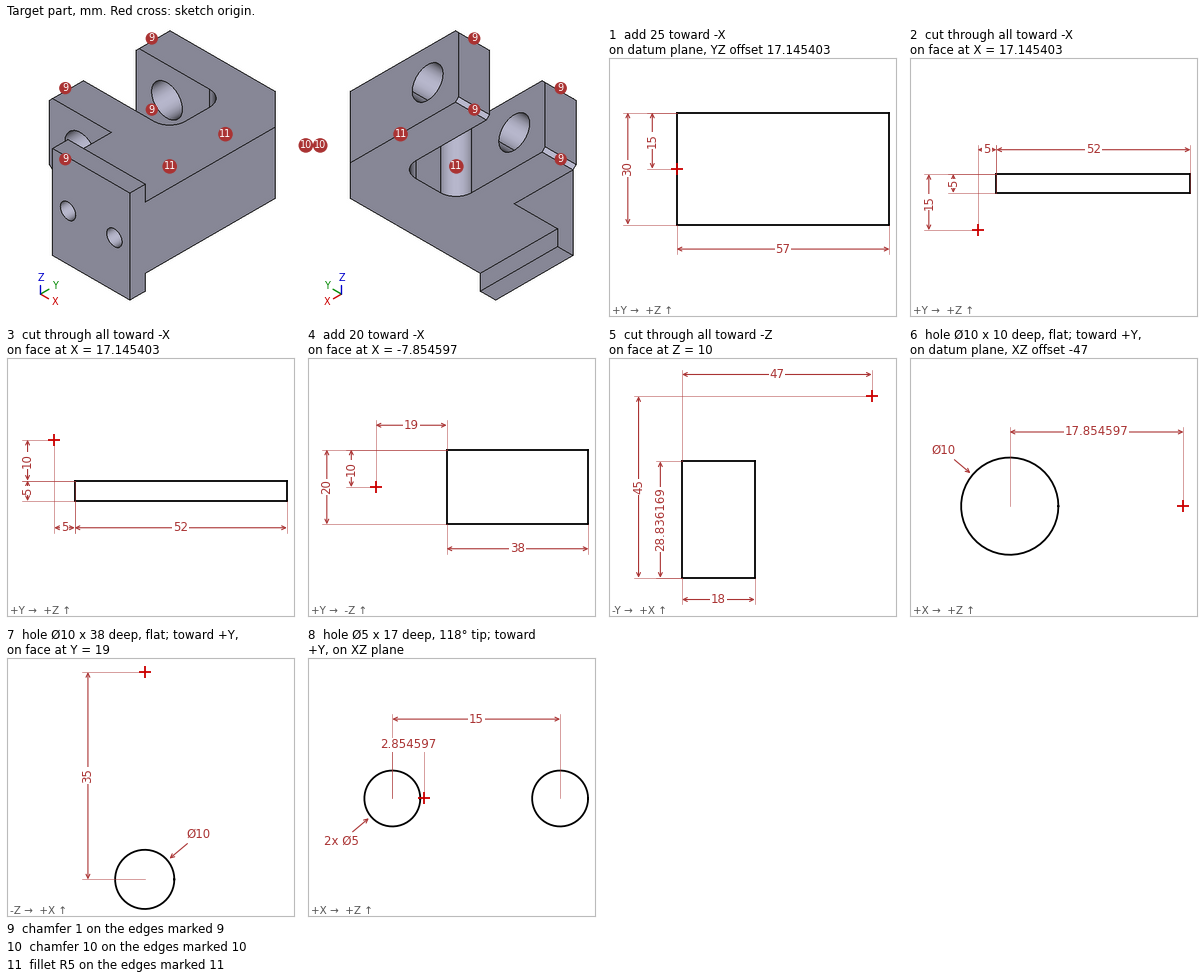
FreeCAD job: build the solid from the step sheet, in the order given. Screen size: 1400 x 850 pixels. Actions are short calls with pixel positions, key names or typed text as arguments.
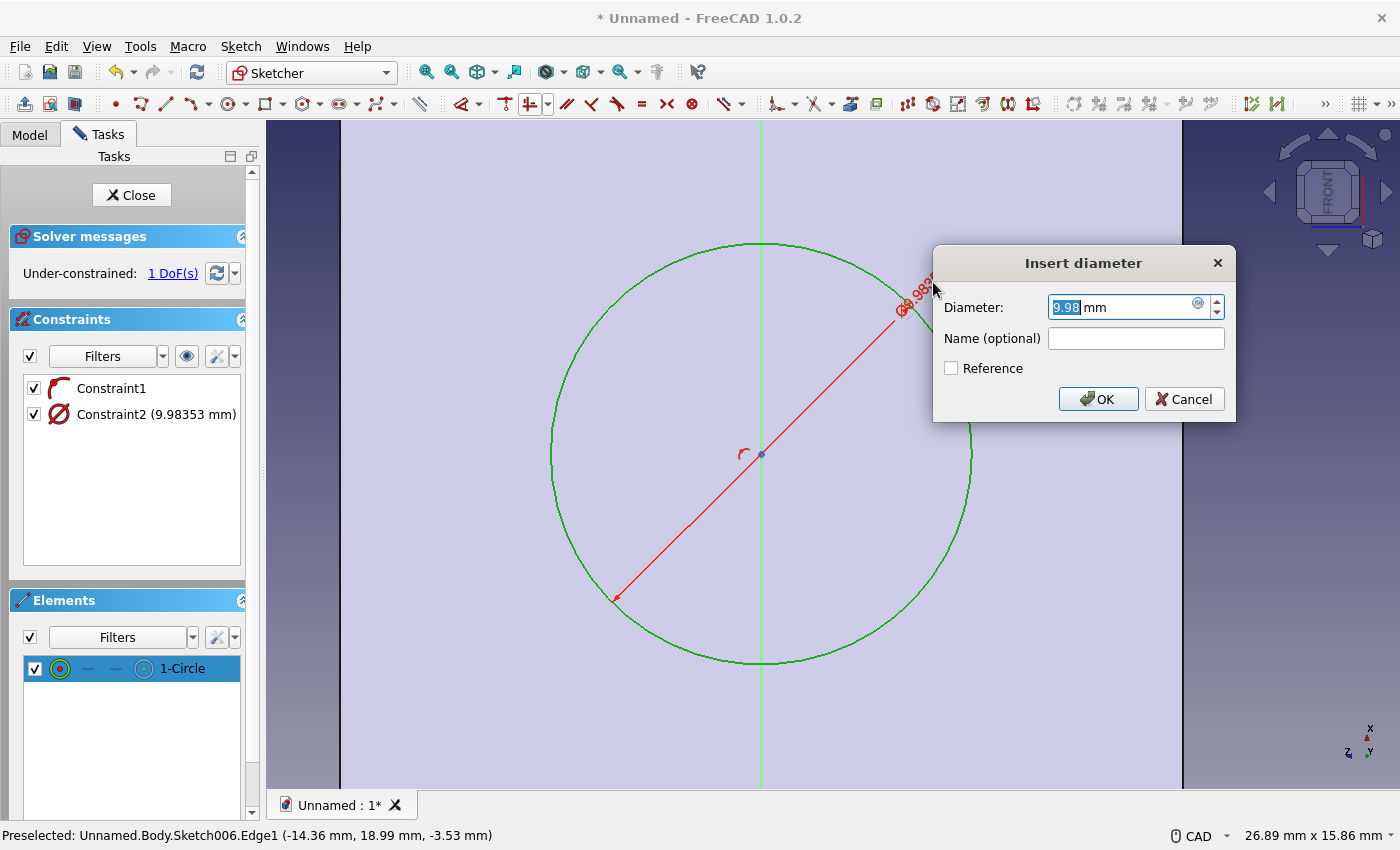
text(10)
key(Return)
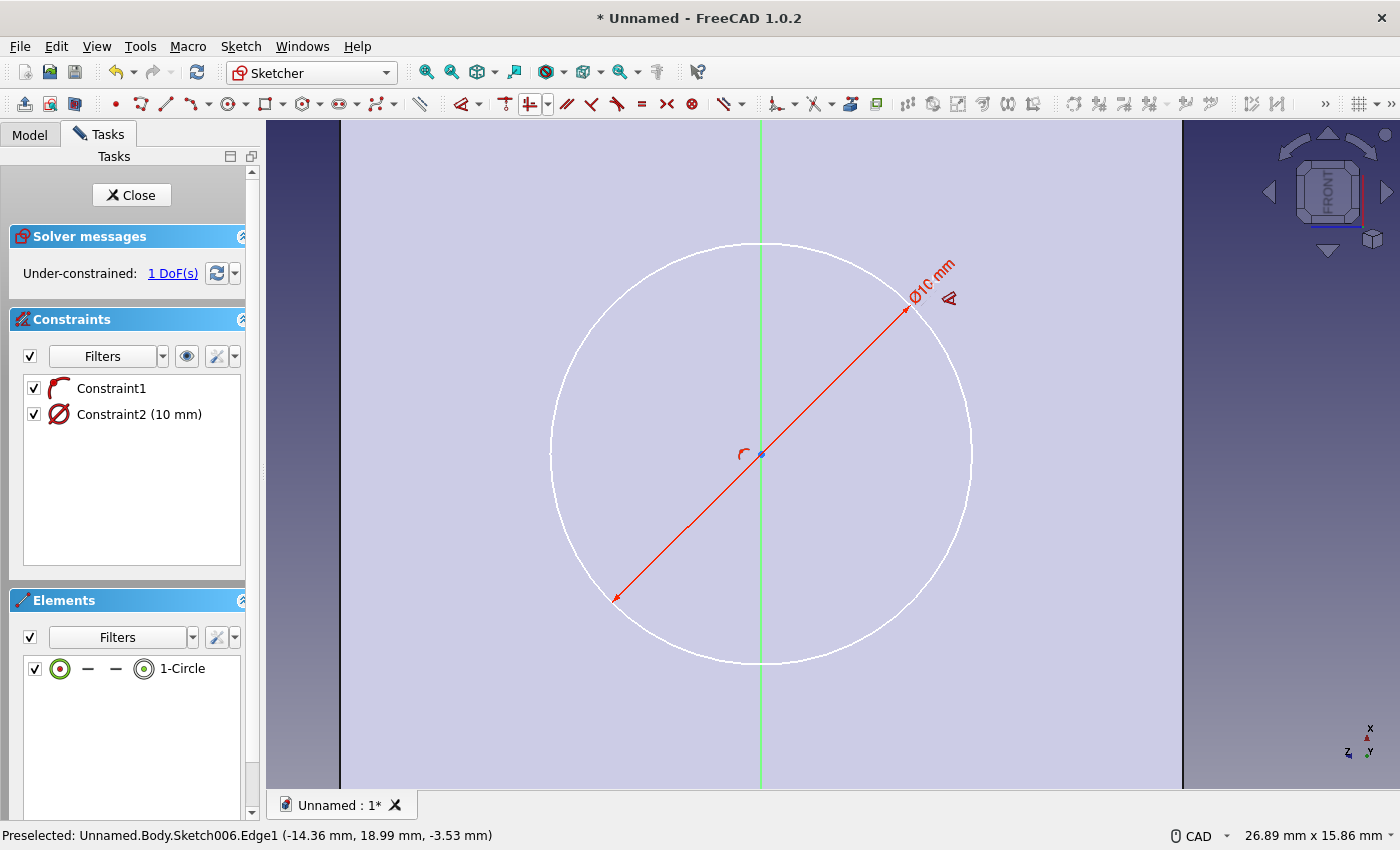
click(761, 454)
click(795, 301)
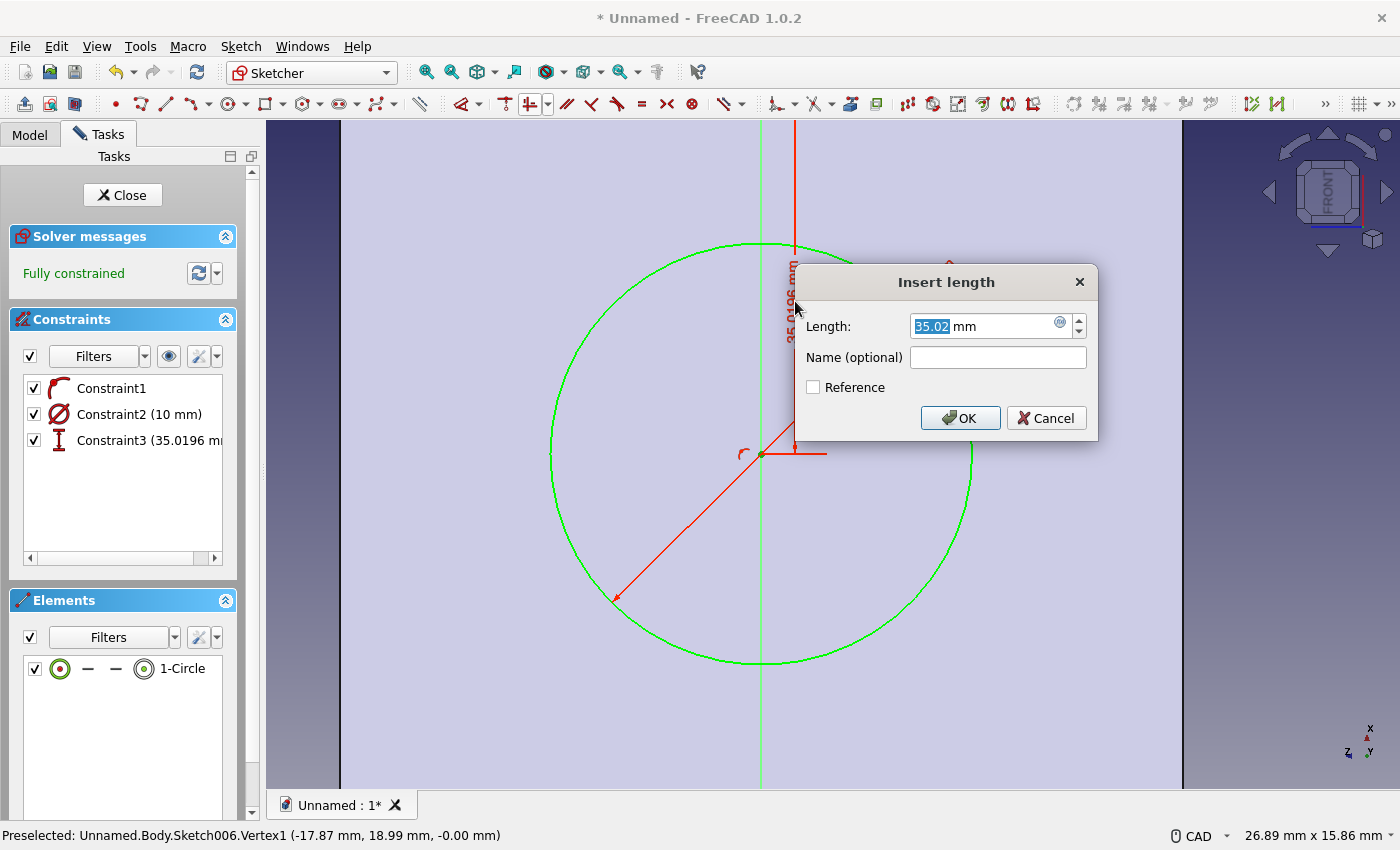
text(35)
key(Return)
key(Escape)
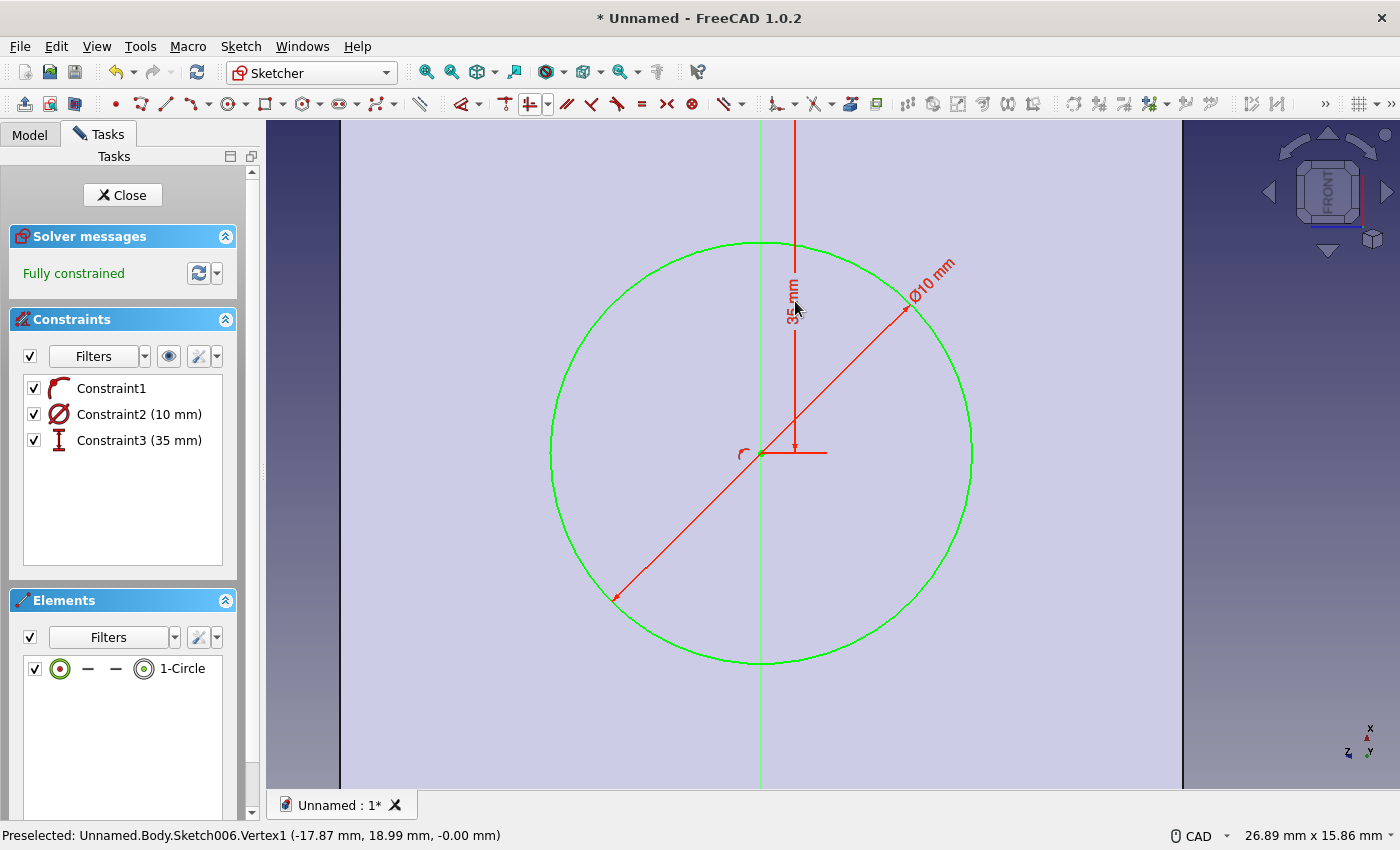
click(123, 195)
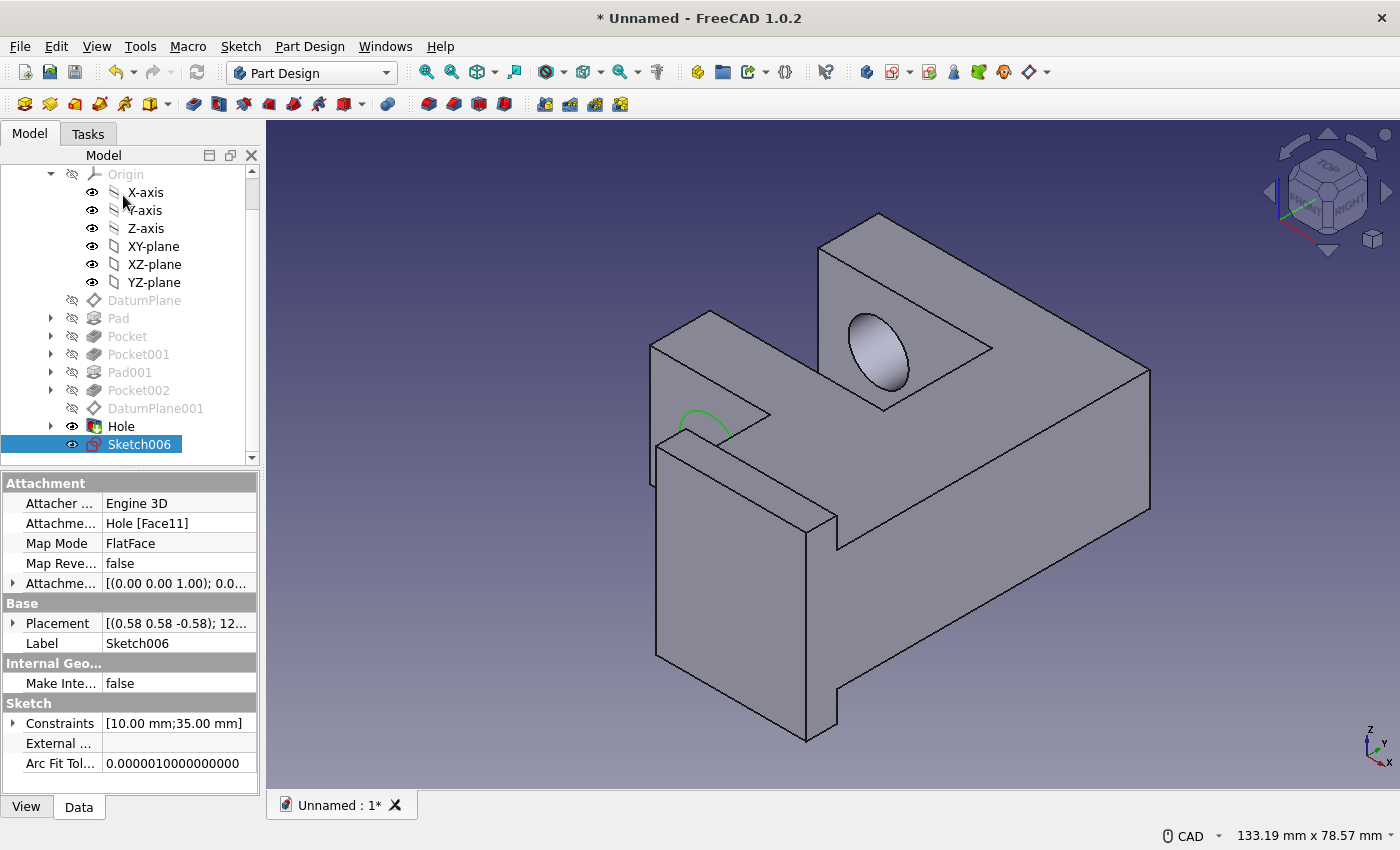
click(219, 104)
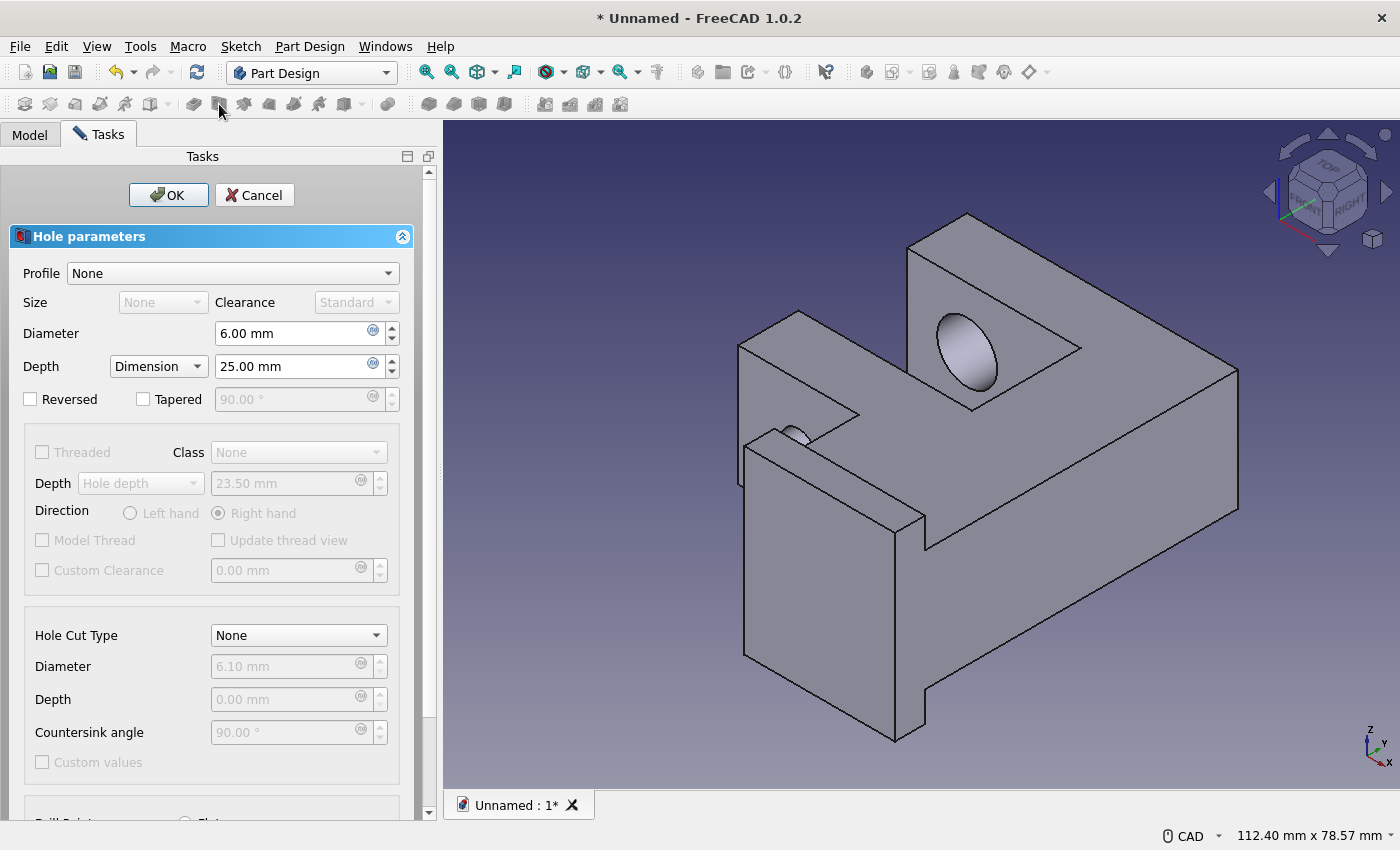
triple_click(300, 334)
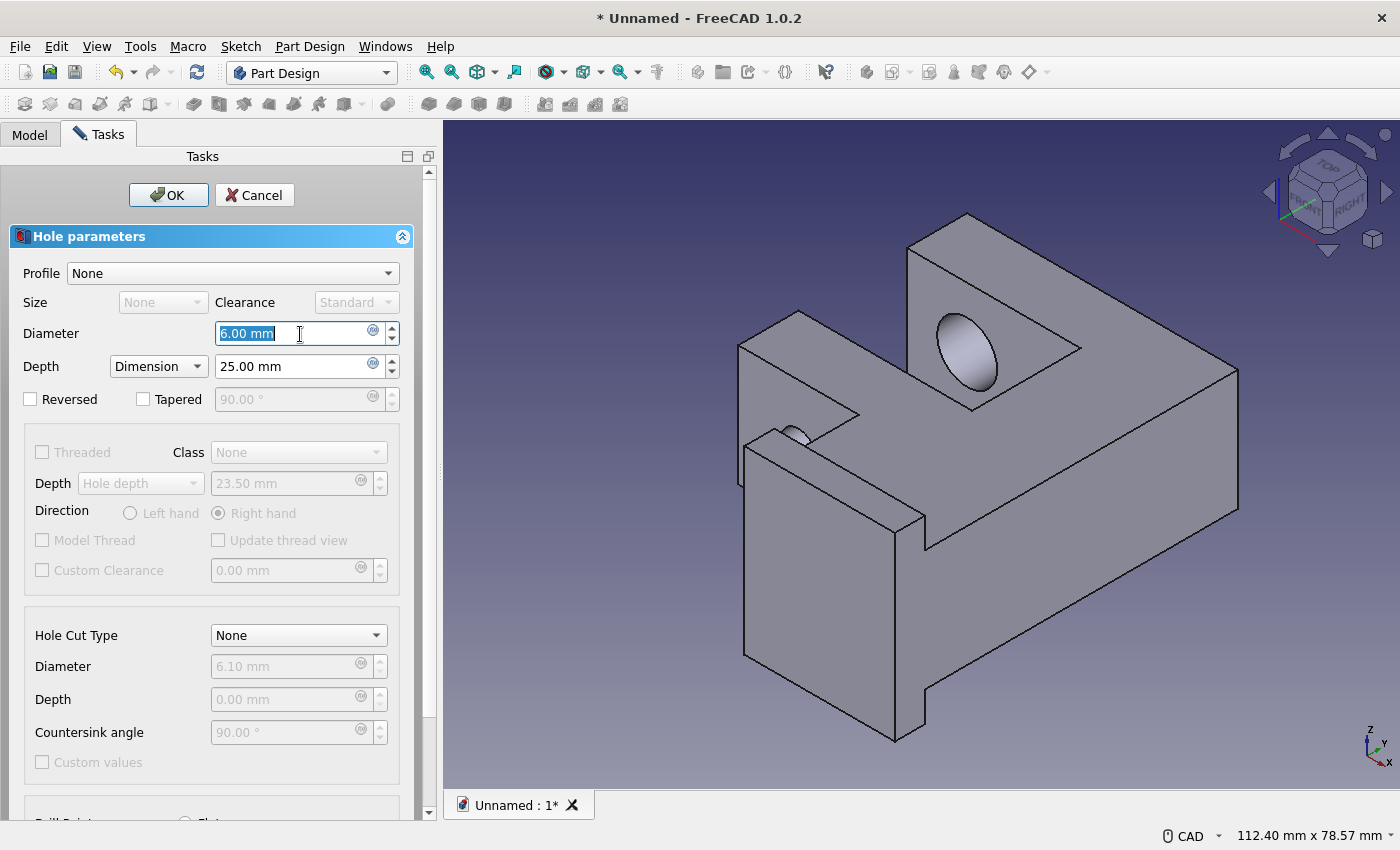
text(10)
key(Tab)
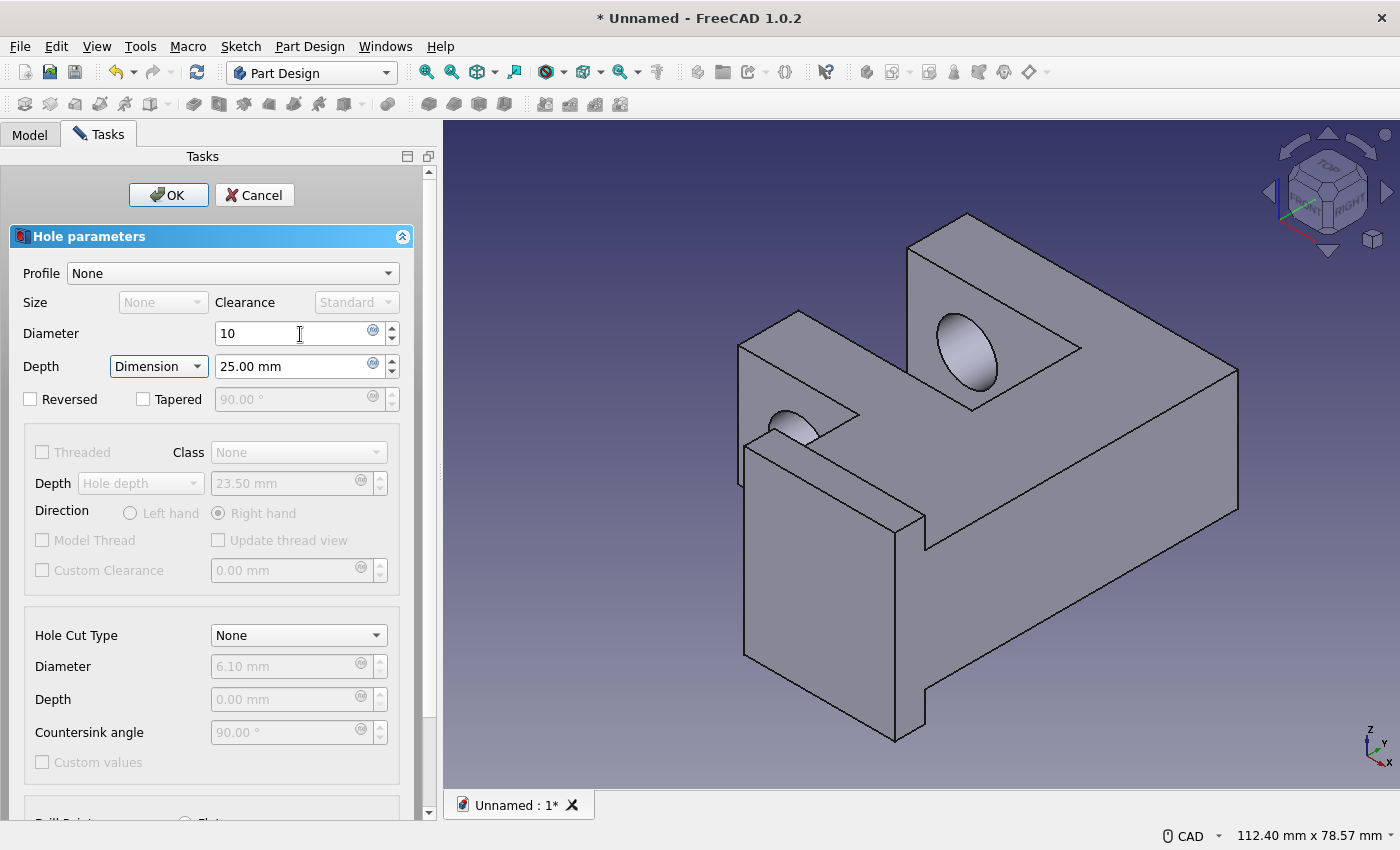
triple_click(300, 366)